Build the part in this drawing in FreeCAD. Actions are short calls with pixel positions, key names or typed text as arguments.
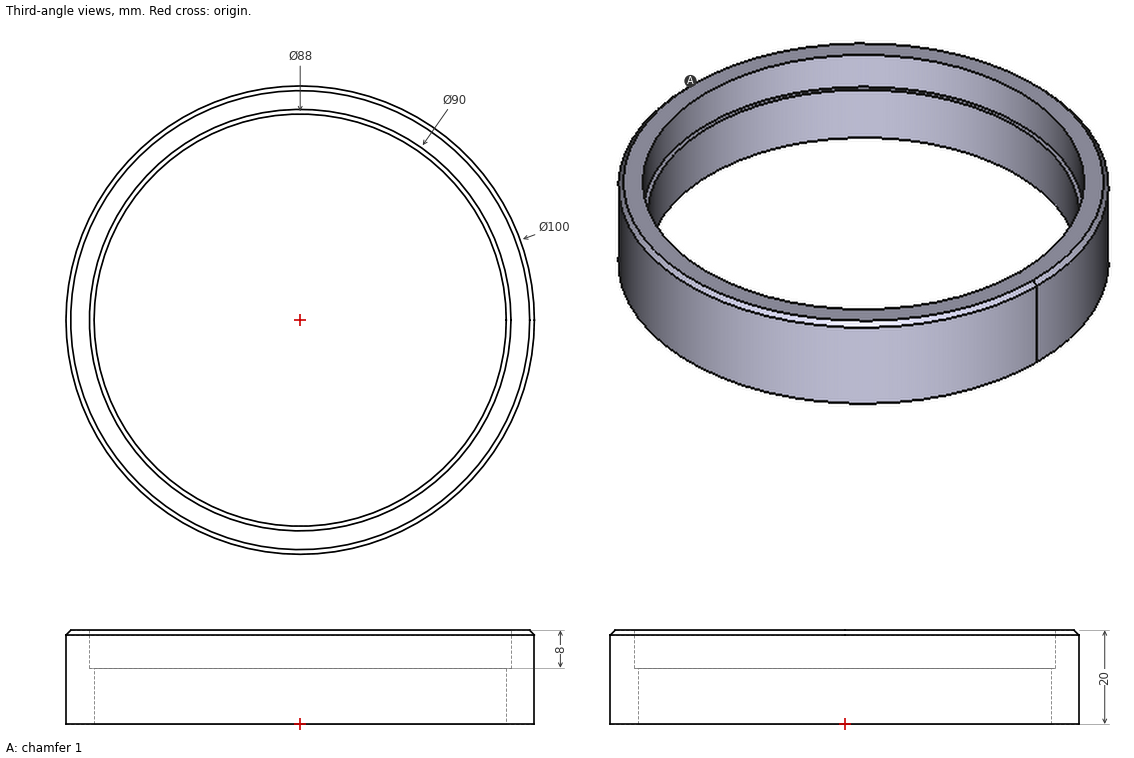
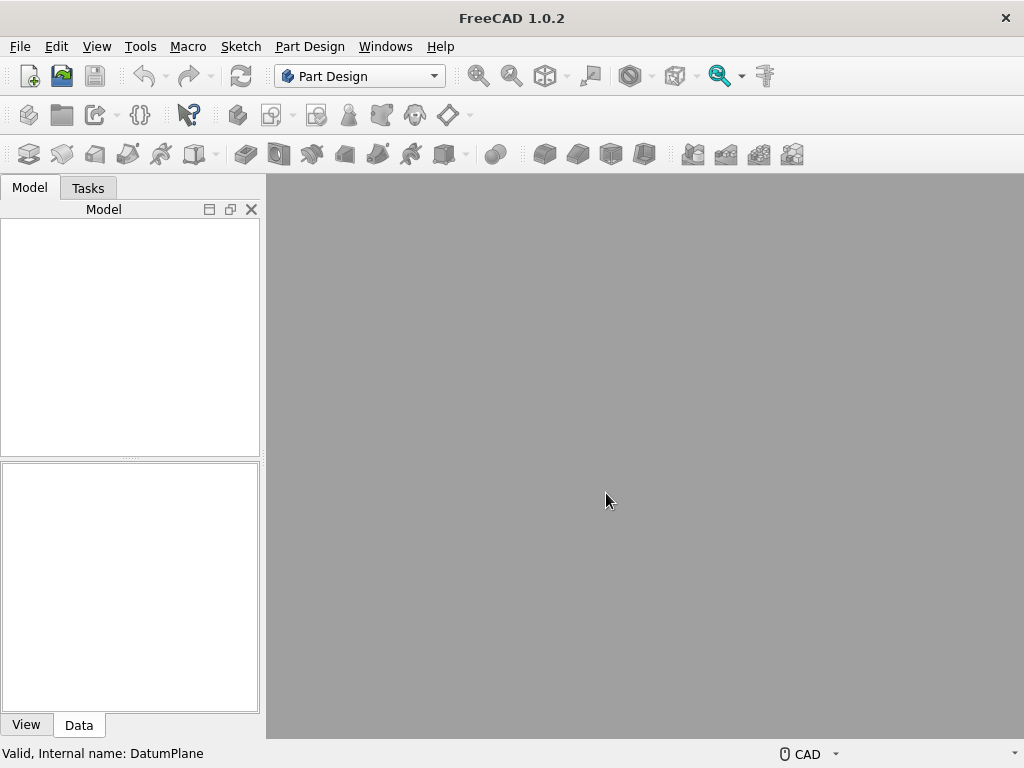
click(29, 76)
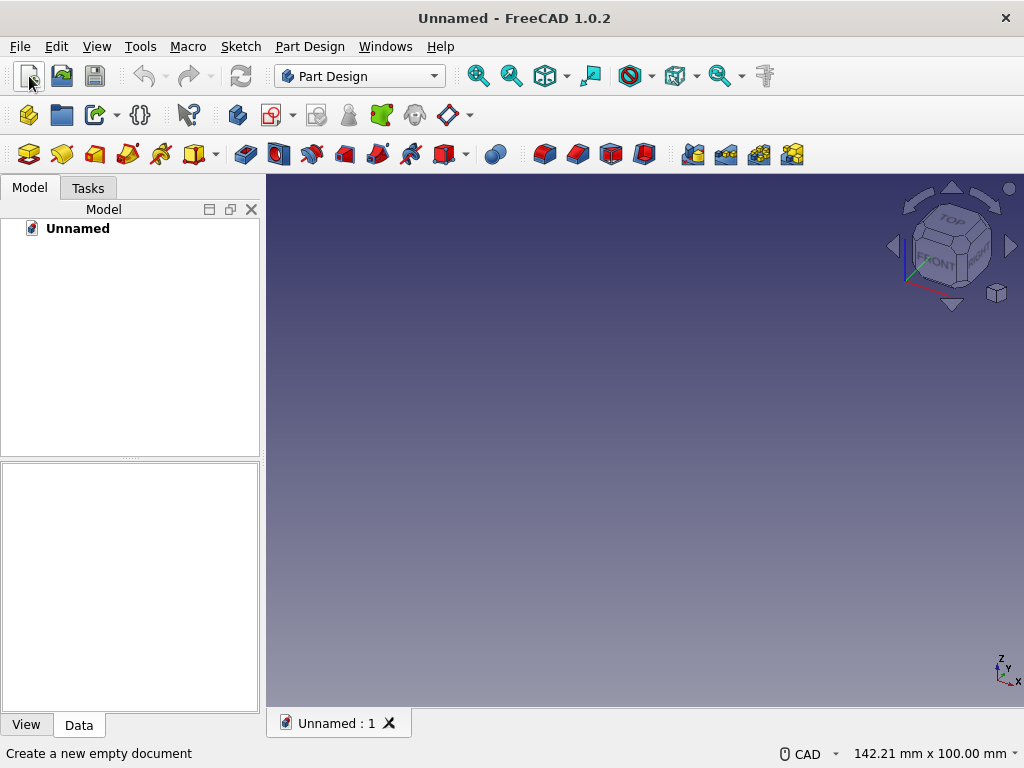
click(270, 116)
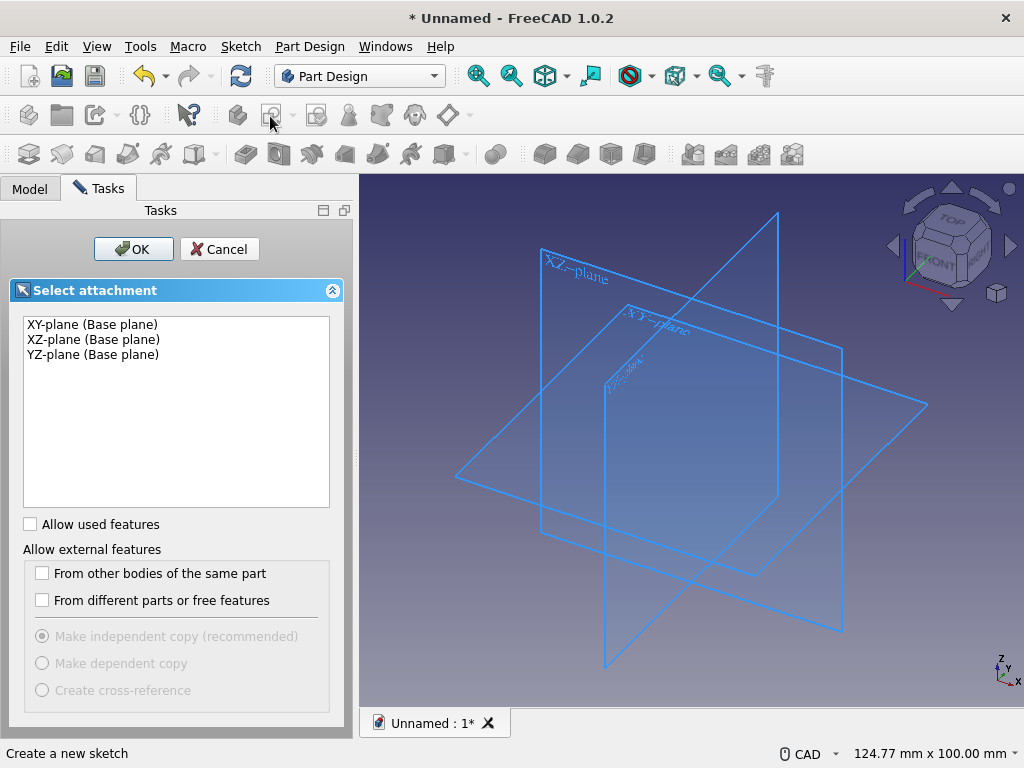
click(84, 324)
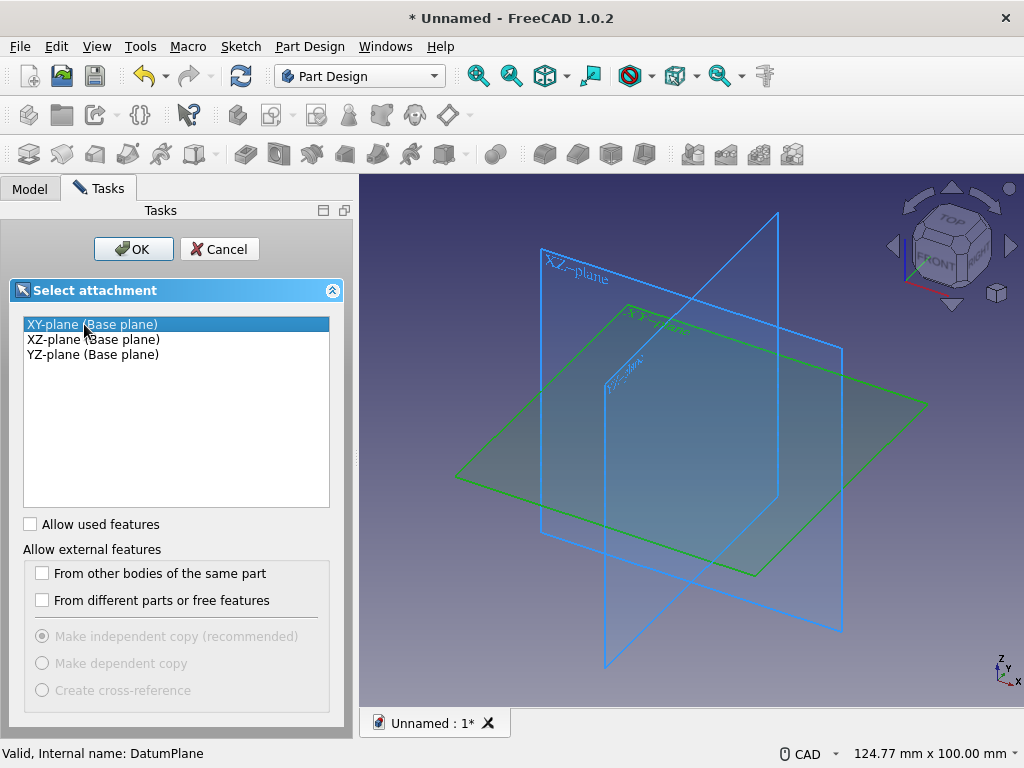
click(134, 249)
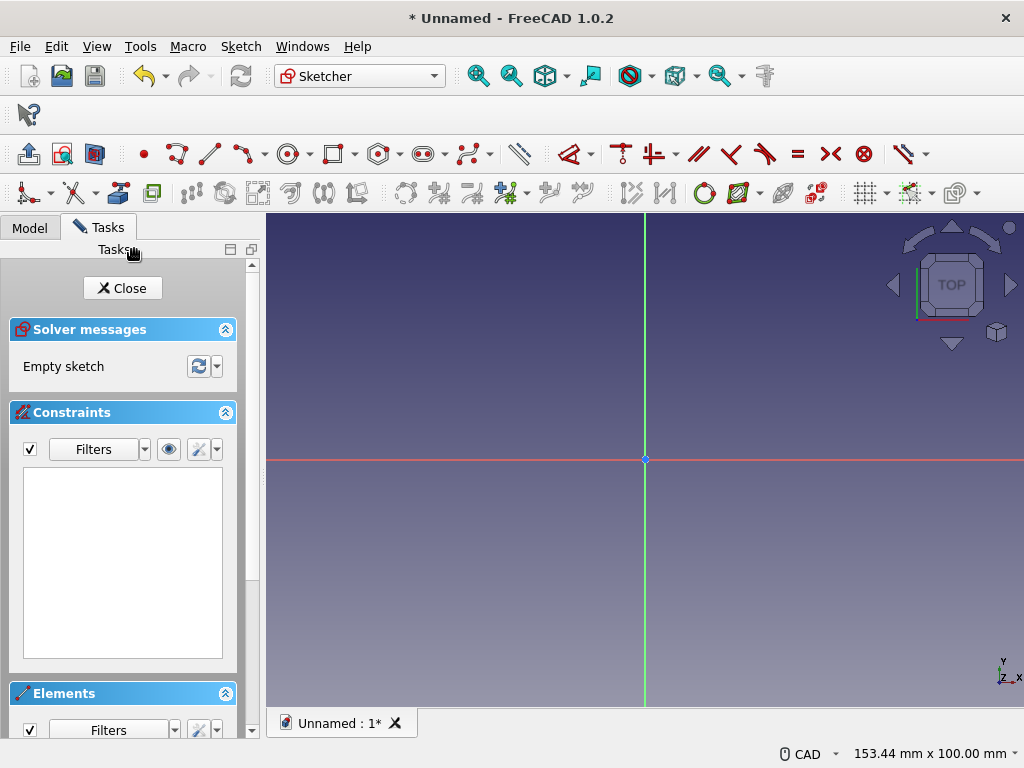
scroll(437, 460, down, 2)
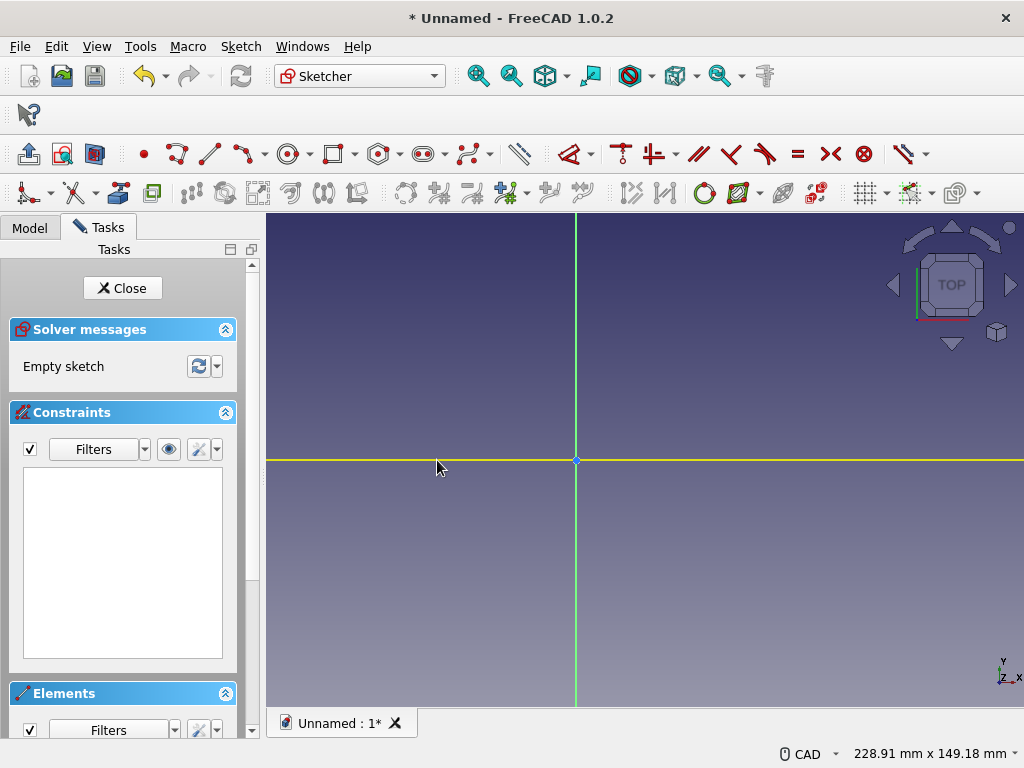
click(288, 154)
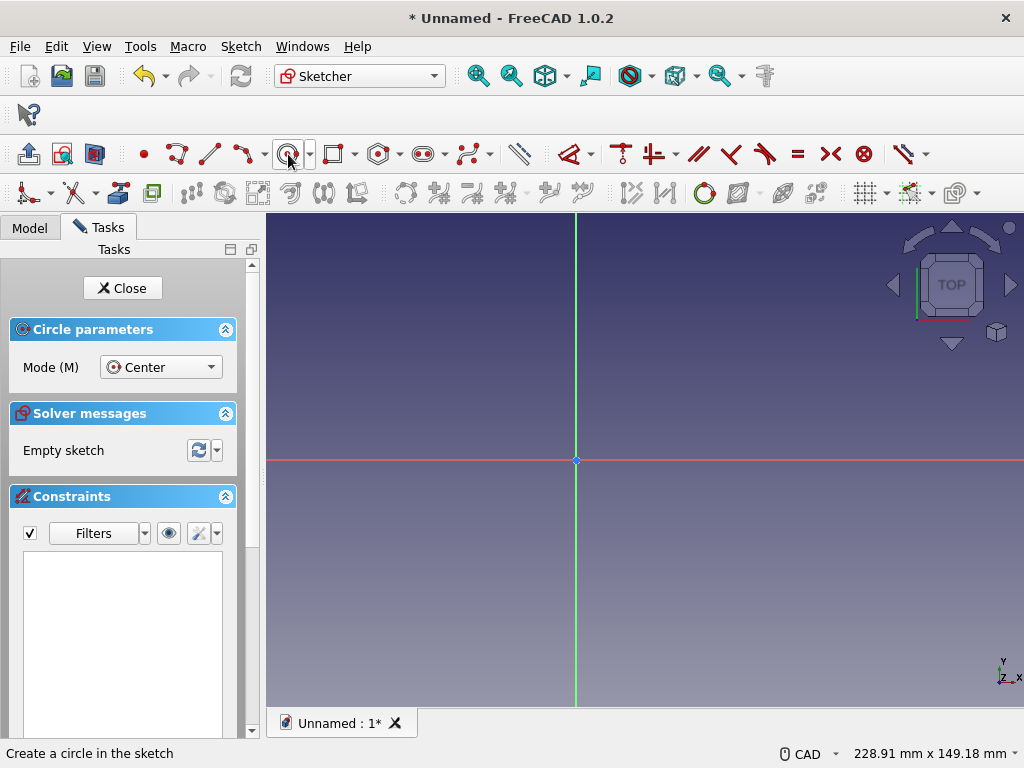
click(577, 460)
move(694, 343)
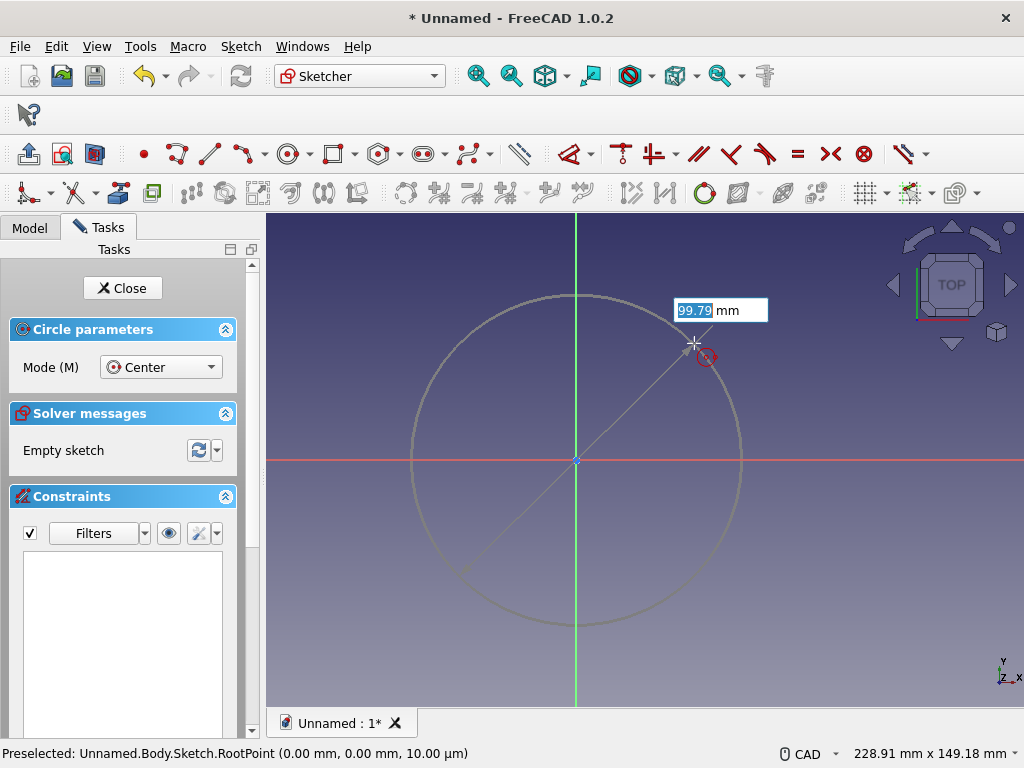
text(100)
key(Return)
key(Escape)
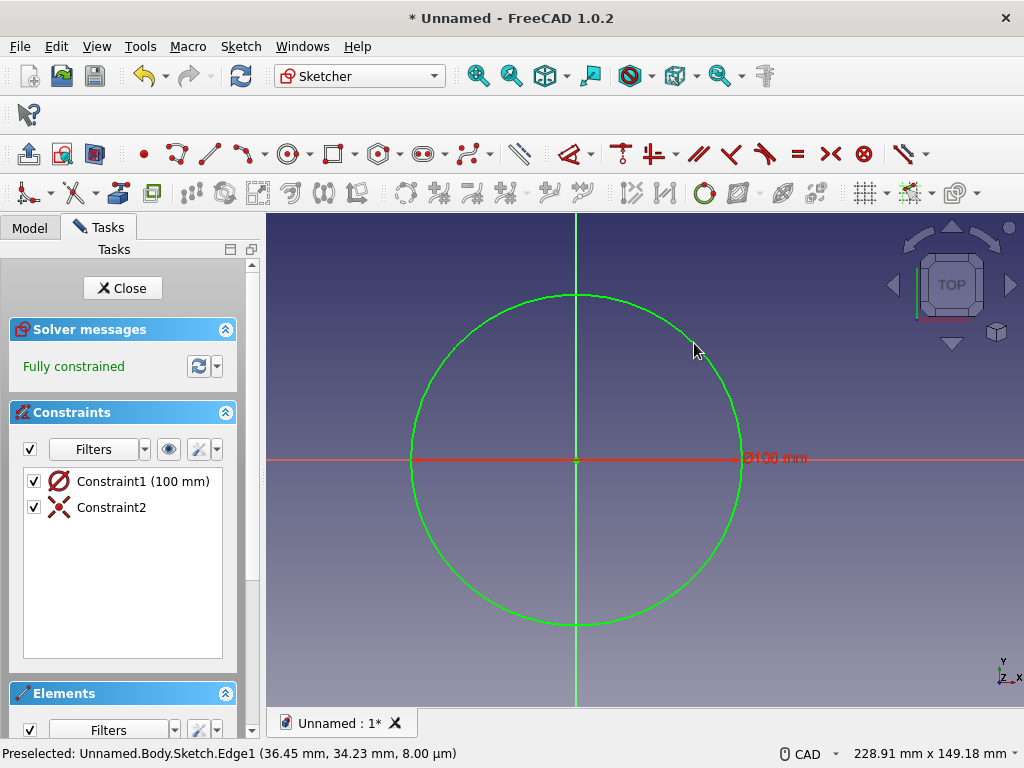
click(123, 288)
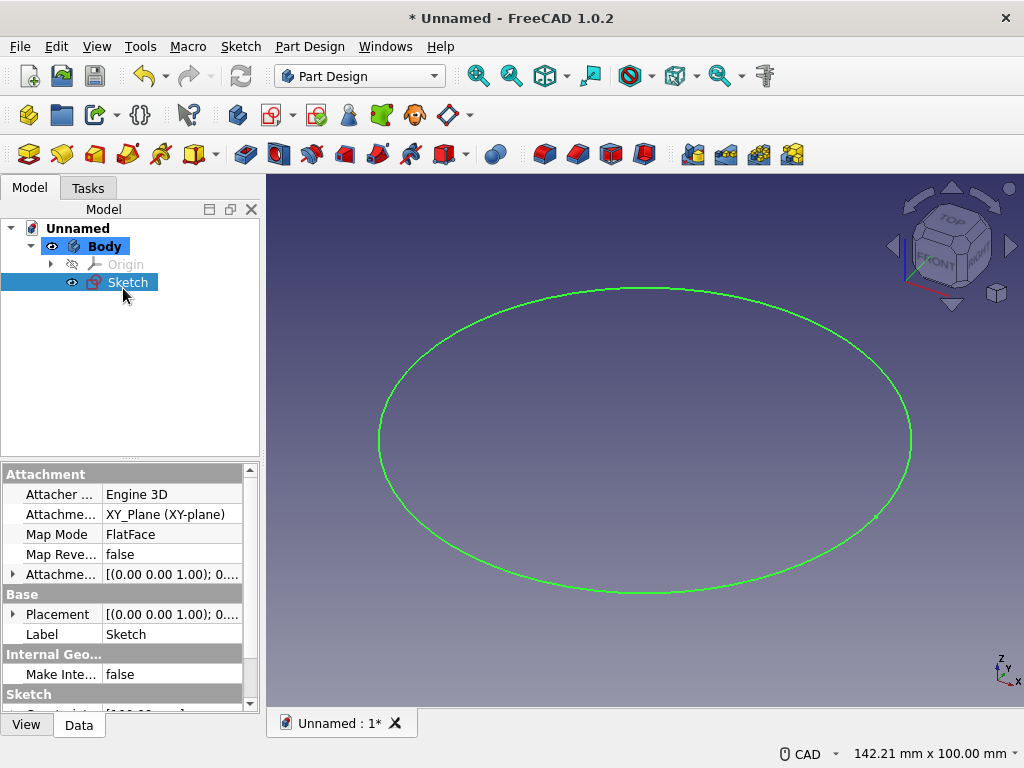
click(29, 154)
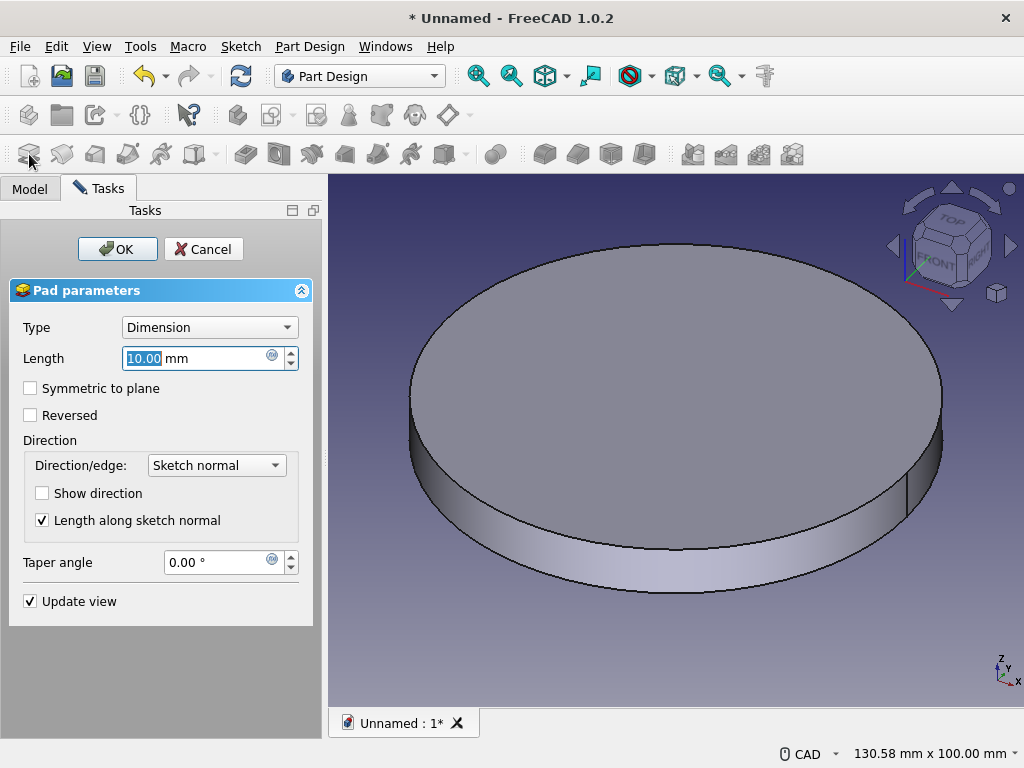
text(20)
key(Tab)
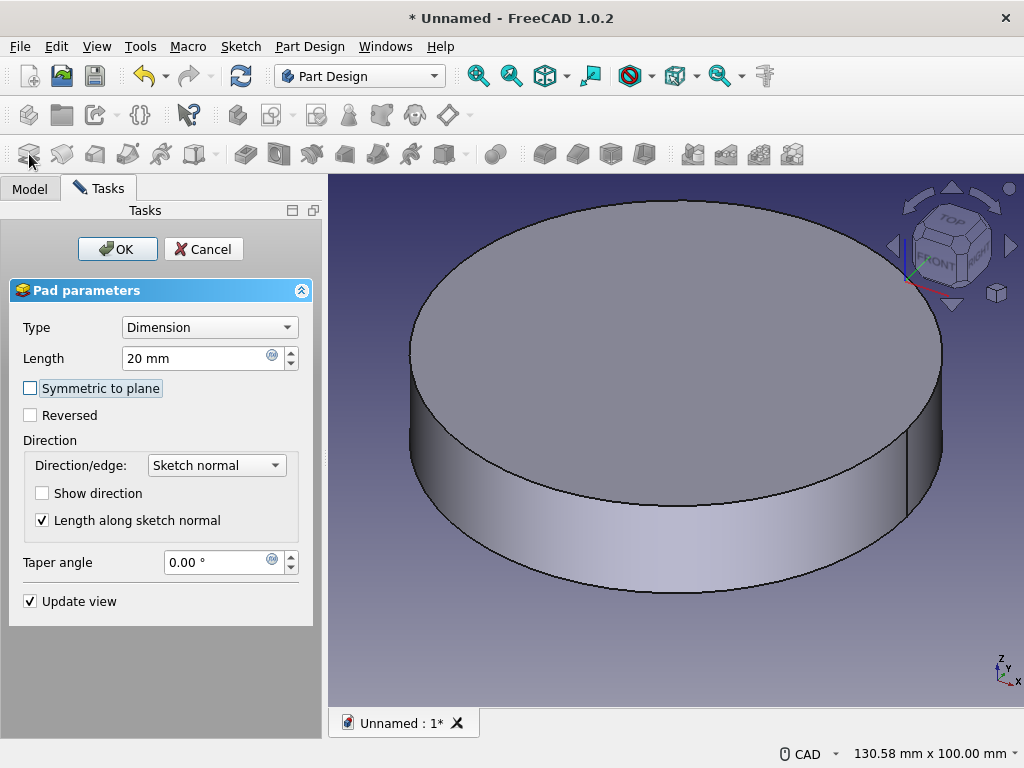
click(118, 249)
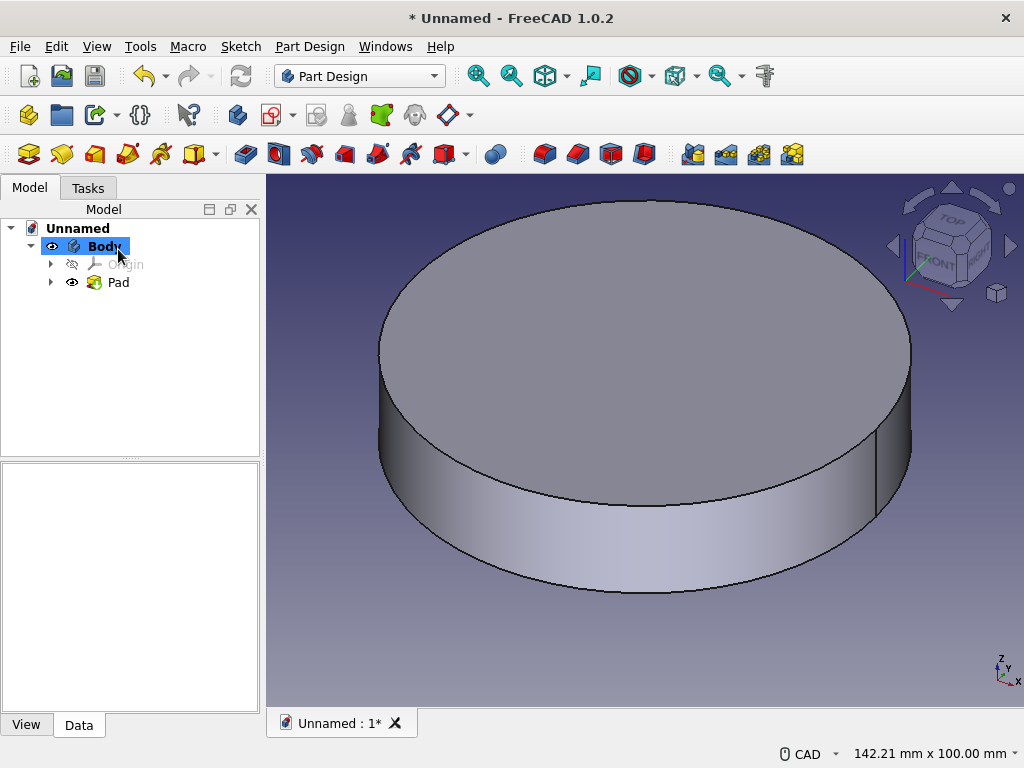
click(479, 76)